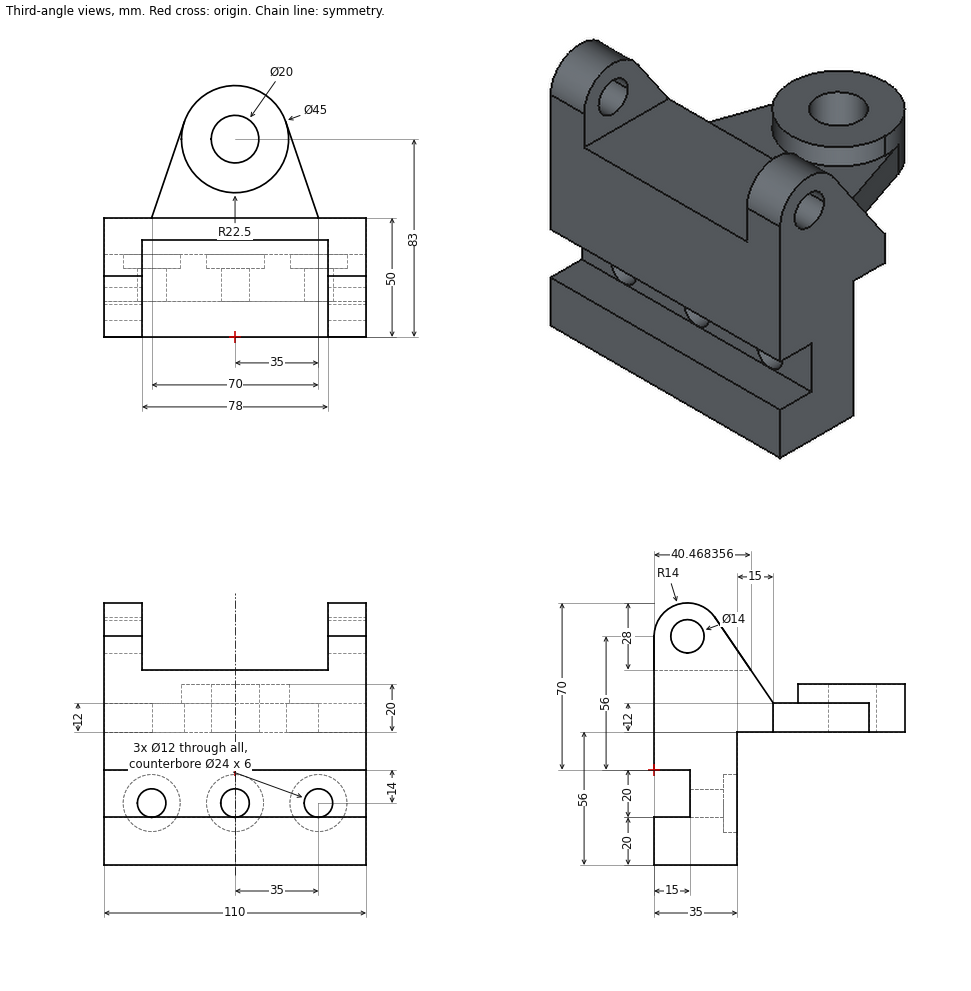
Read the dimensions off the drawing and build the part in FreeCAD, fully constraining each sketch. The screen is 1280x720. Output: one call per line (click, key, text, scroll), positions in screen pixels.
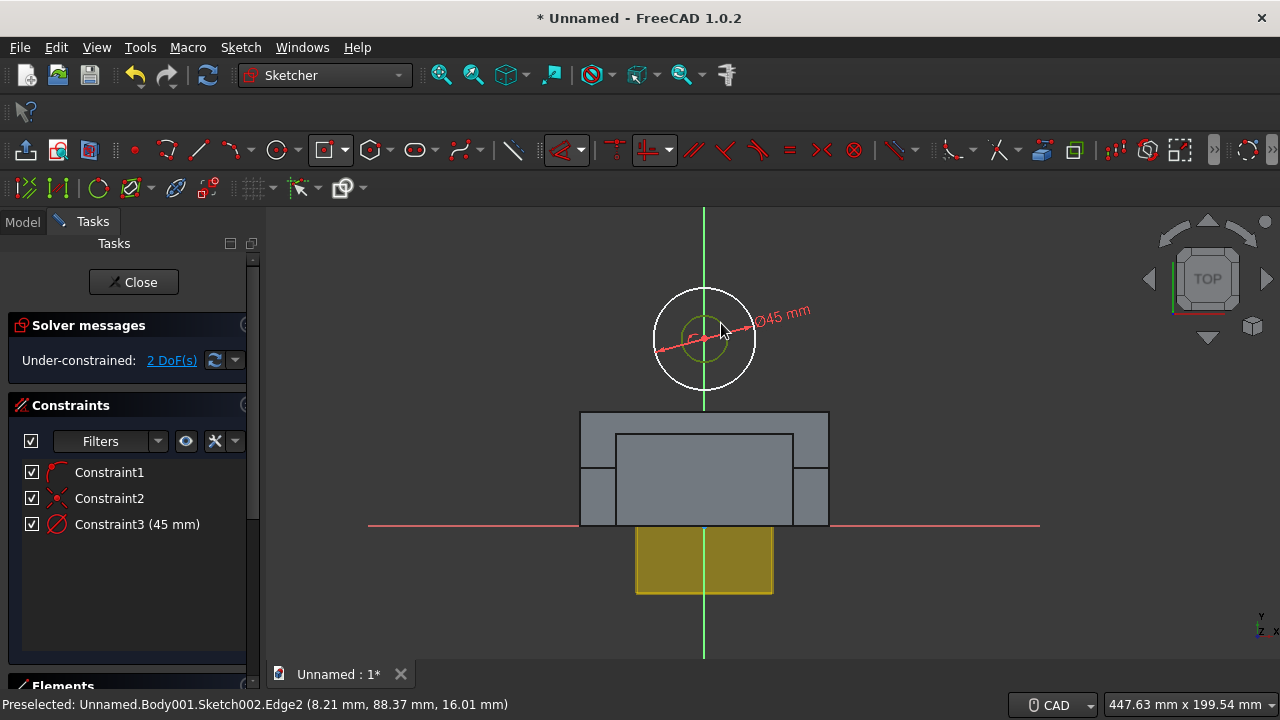
key(k)
key(o)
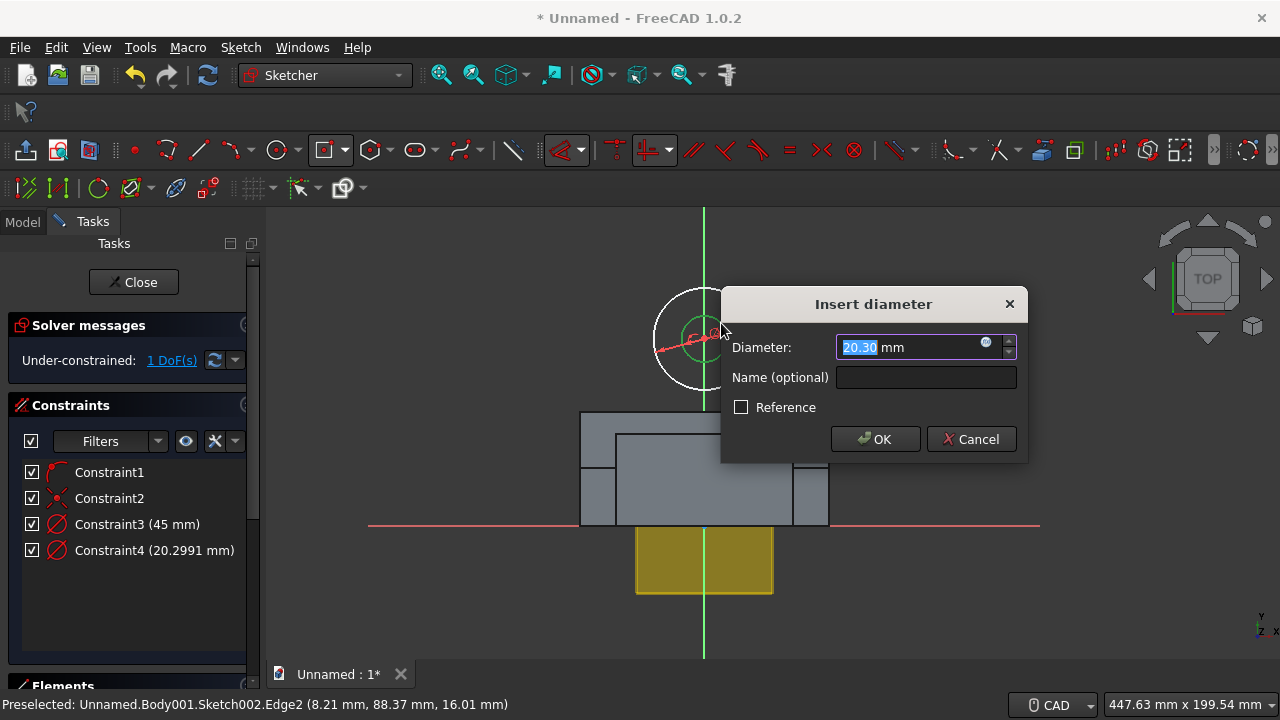
text(20)
key(Return)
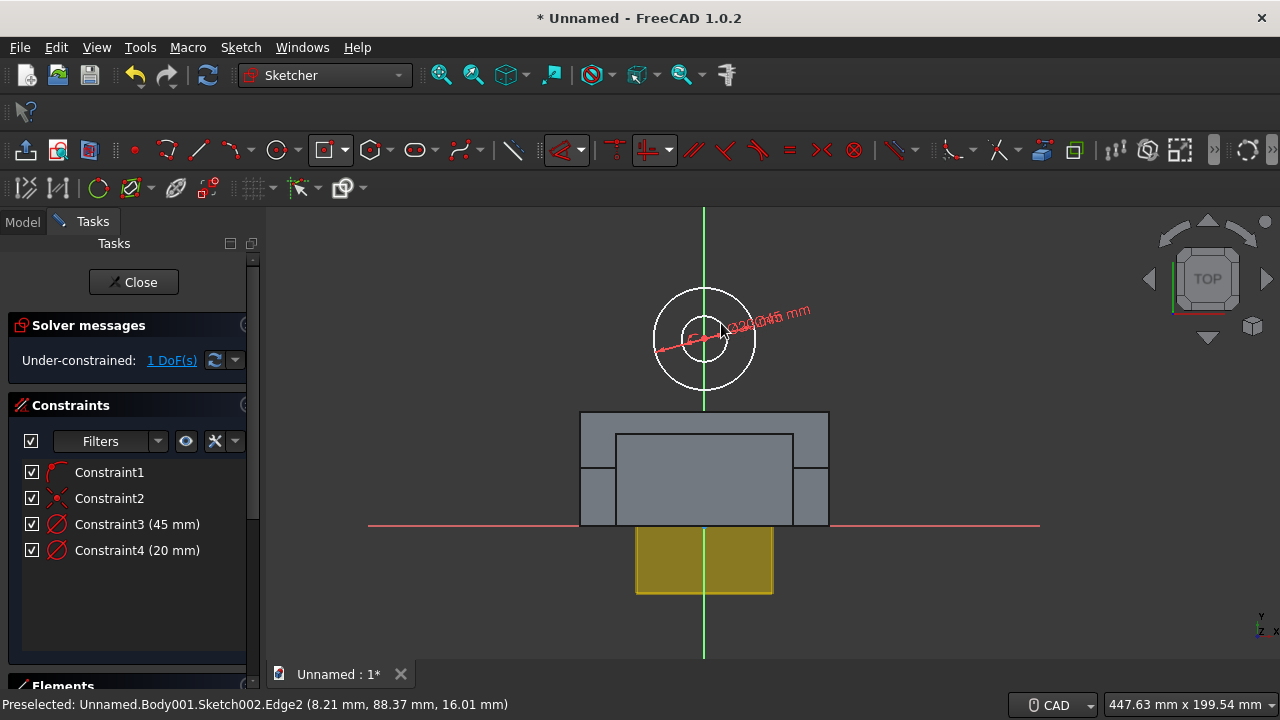
click(704, 339)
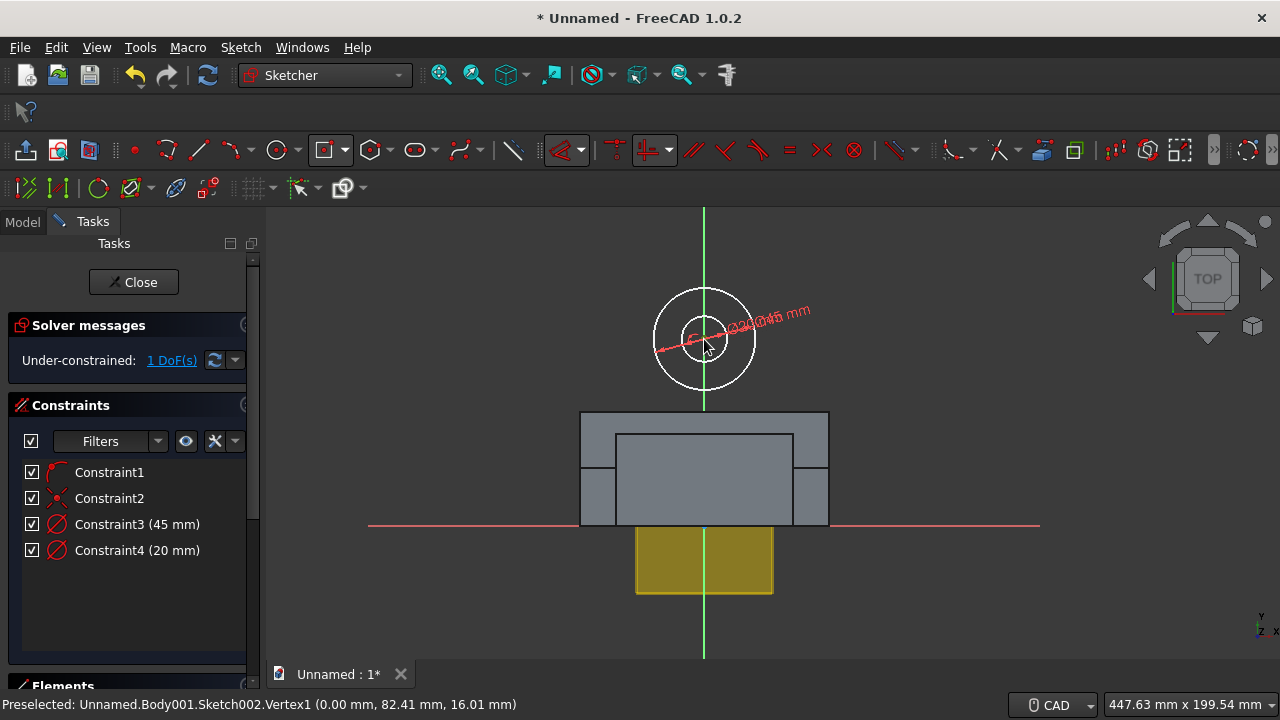
key(i)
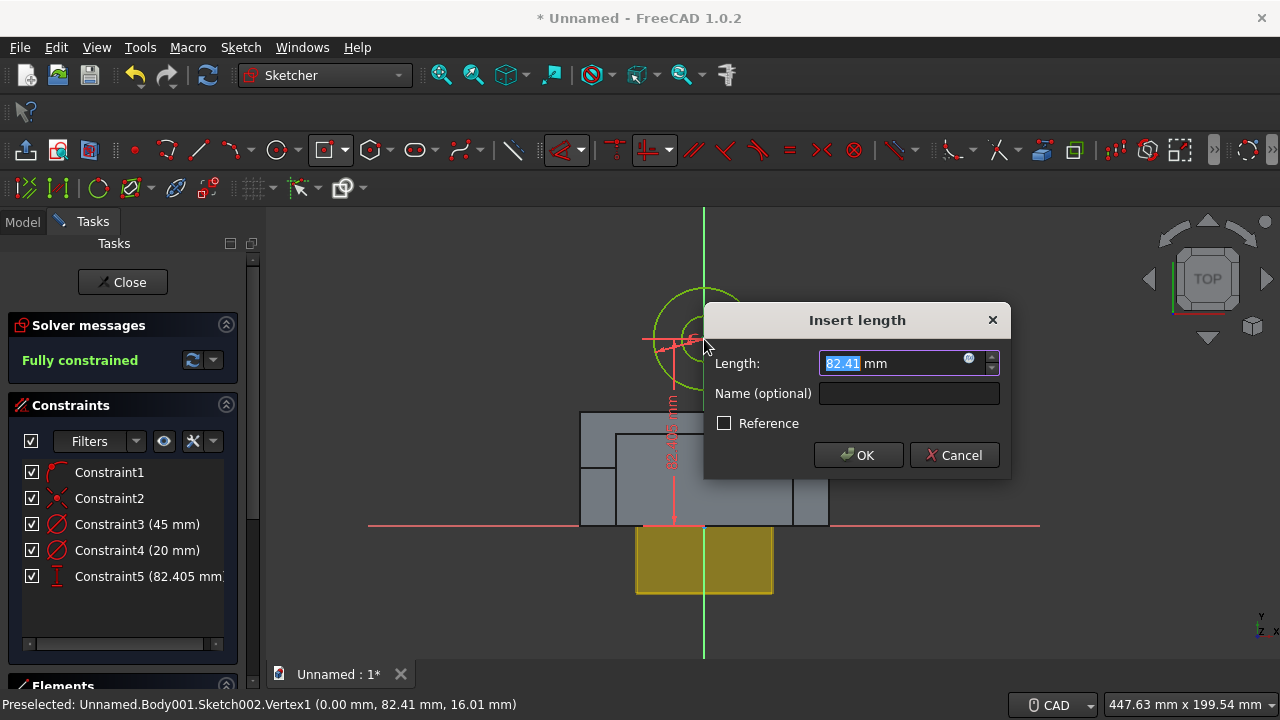
text(83)
key(Return)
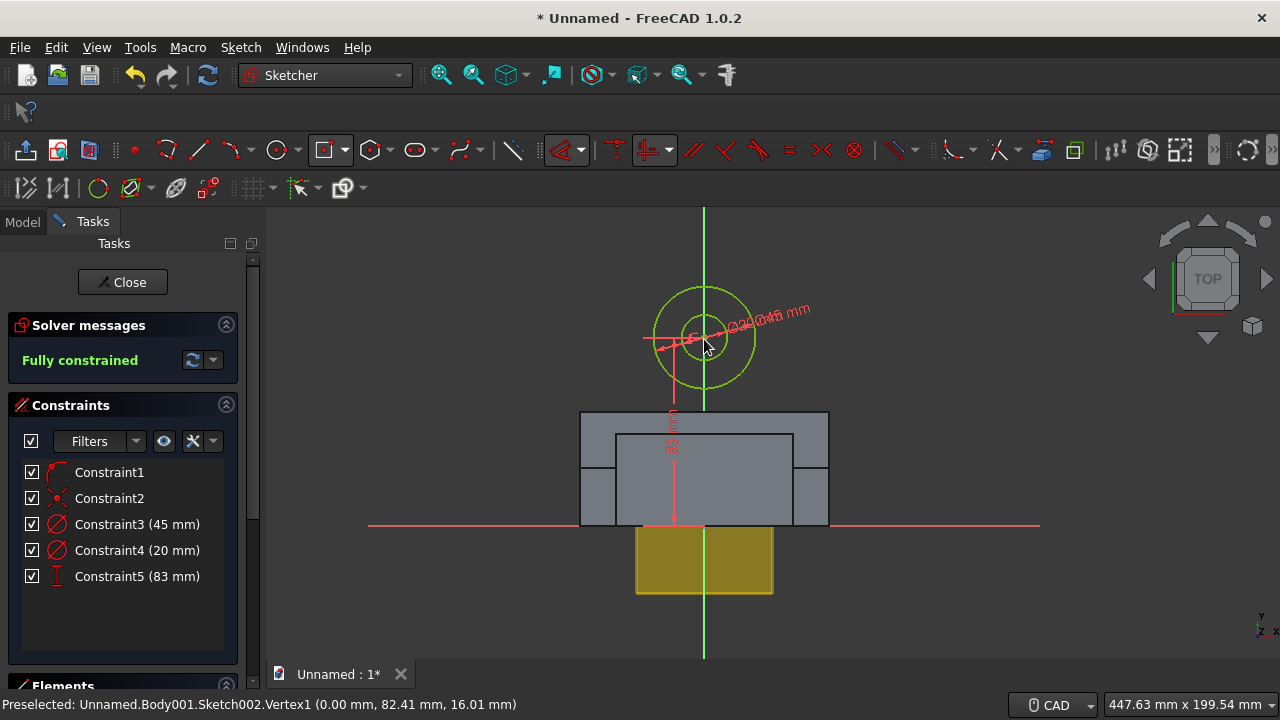
click(123, 282)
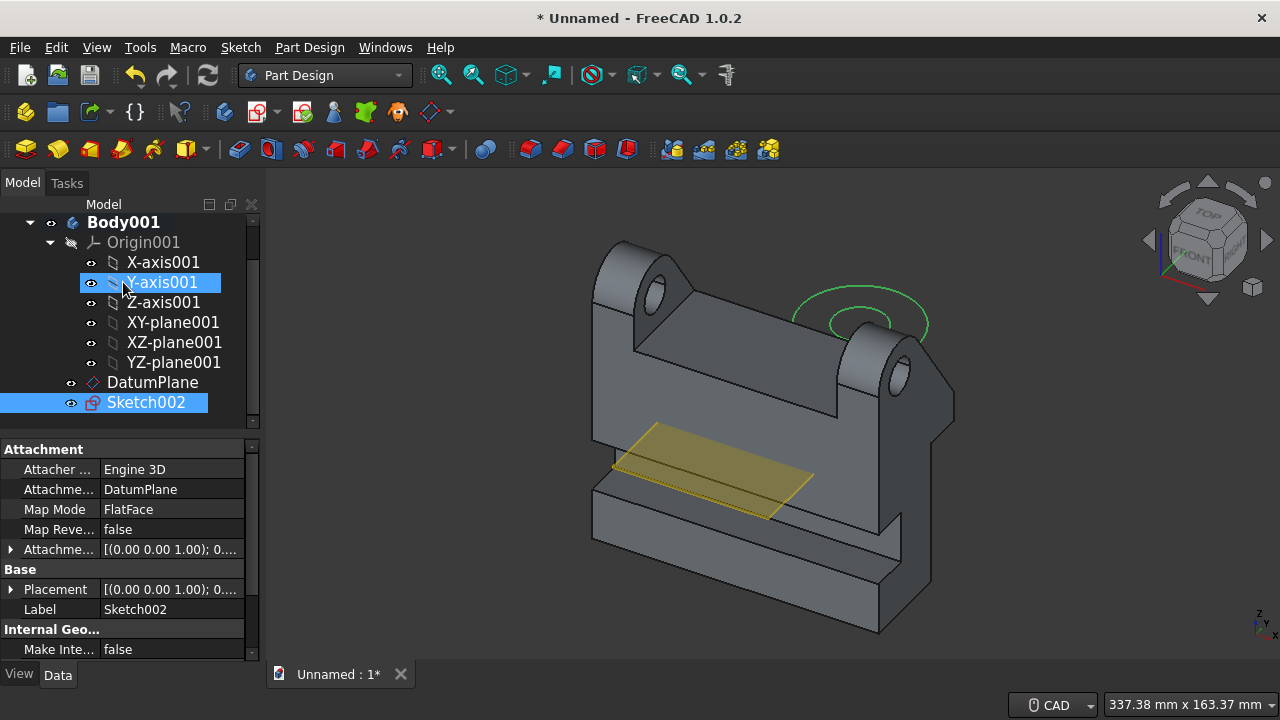
click(26, 150)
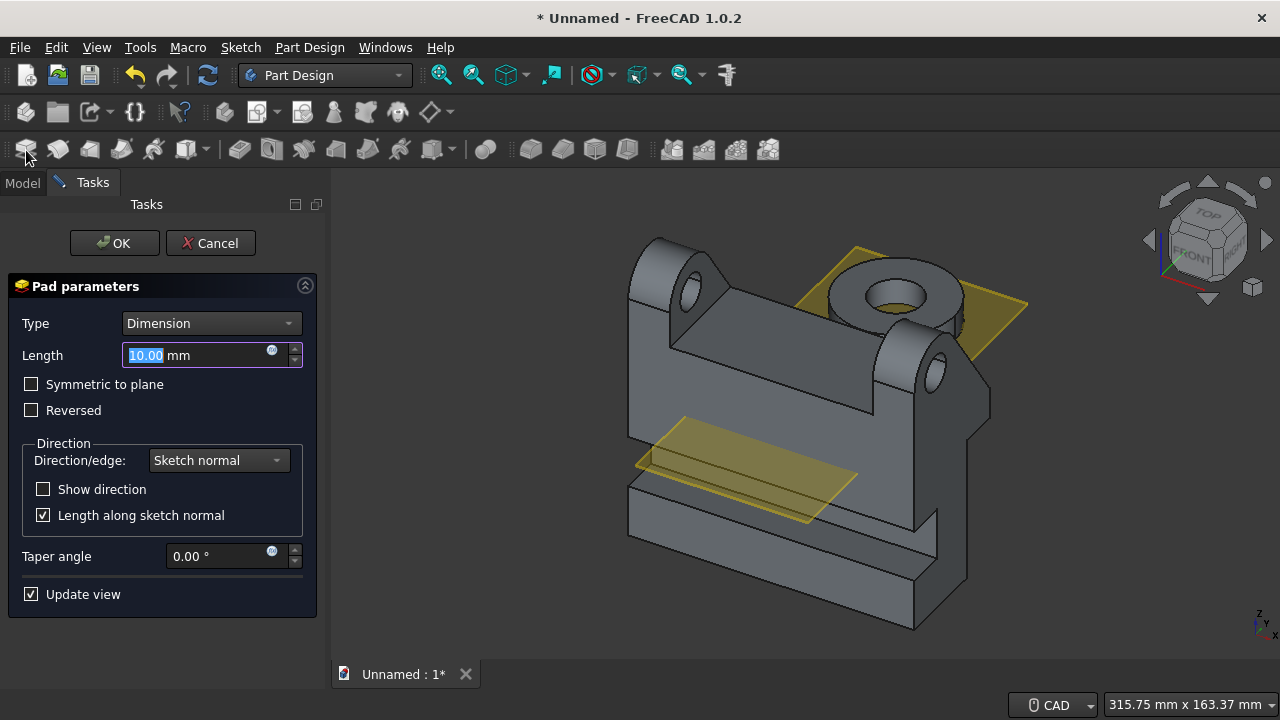
text(20)
key(Tab)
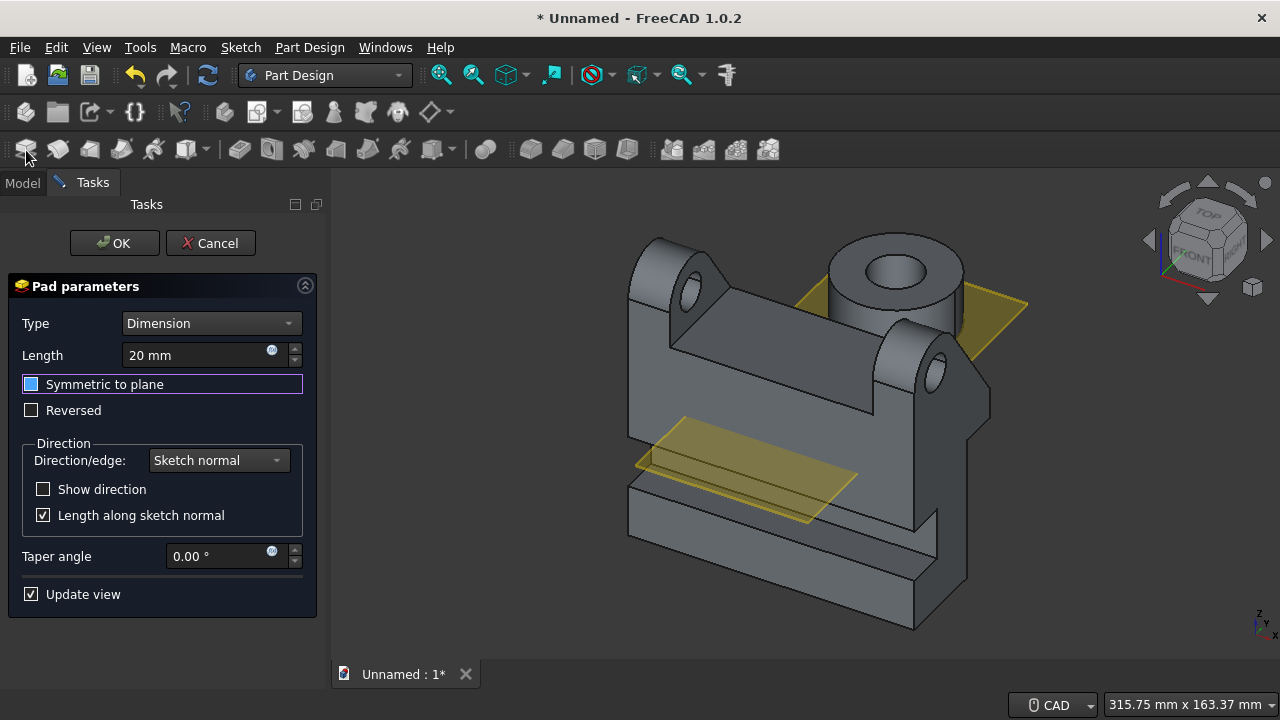
click(115, 243)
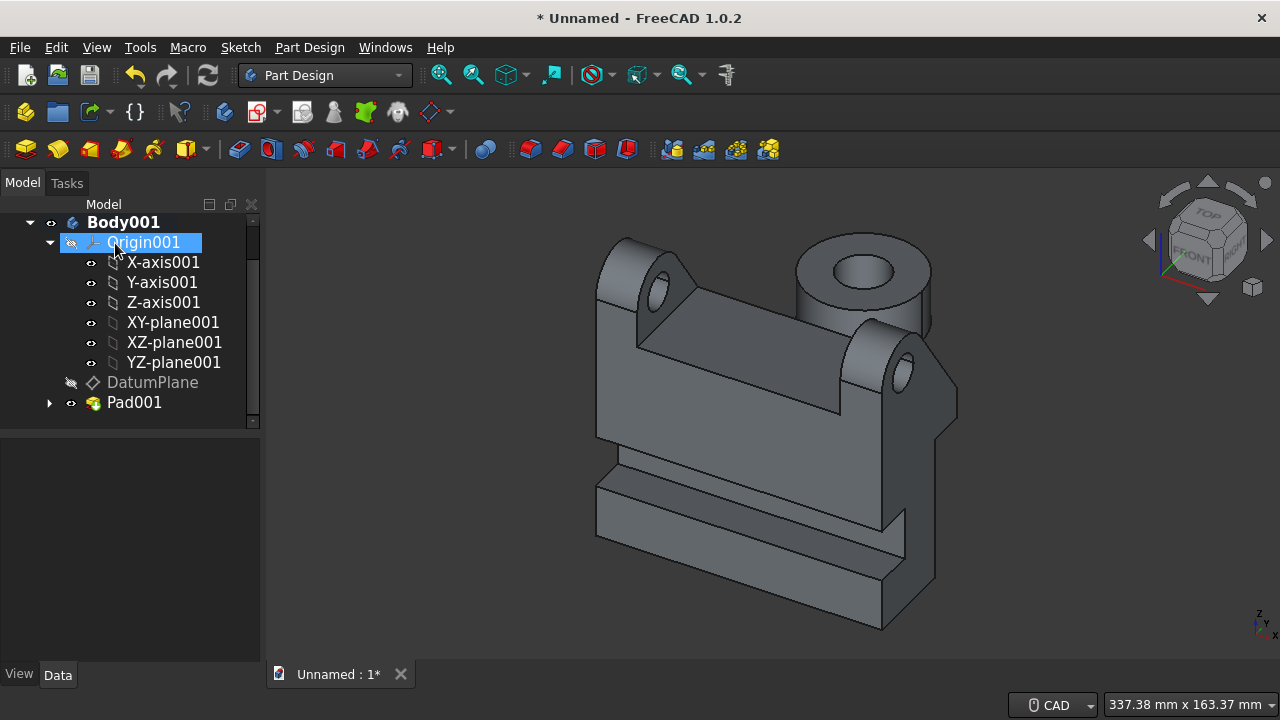
click(442, 76)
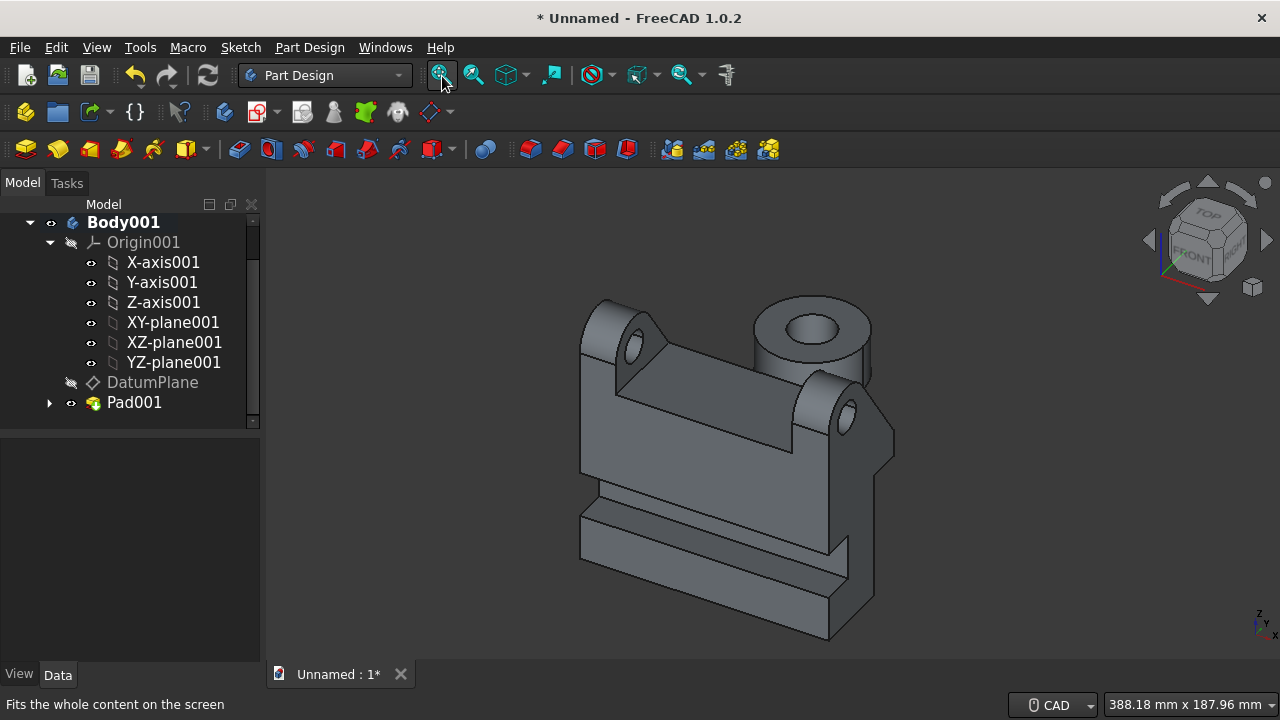
scroll(120, 318, down, 3)